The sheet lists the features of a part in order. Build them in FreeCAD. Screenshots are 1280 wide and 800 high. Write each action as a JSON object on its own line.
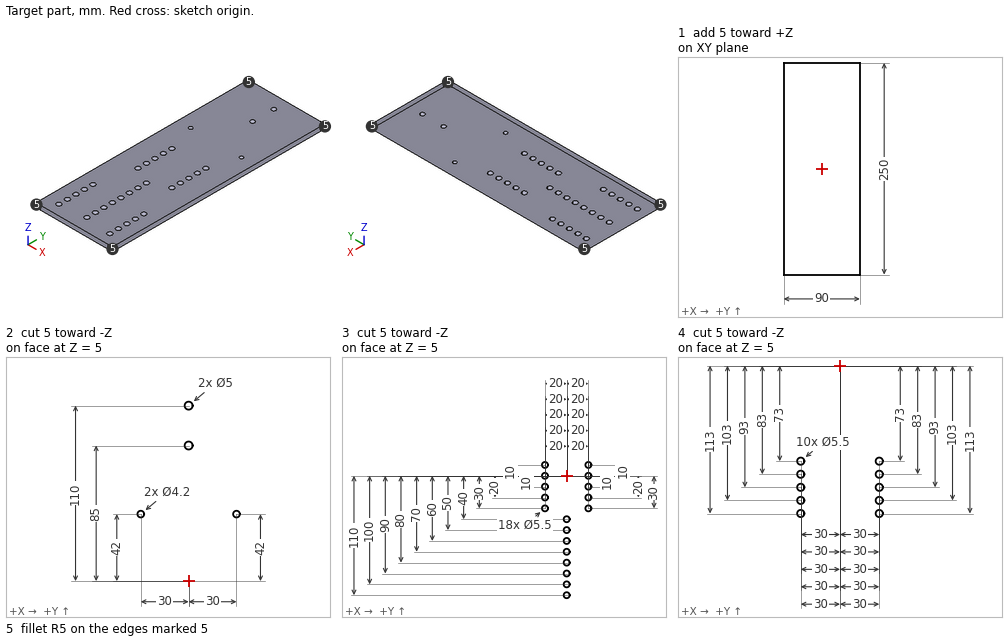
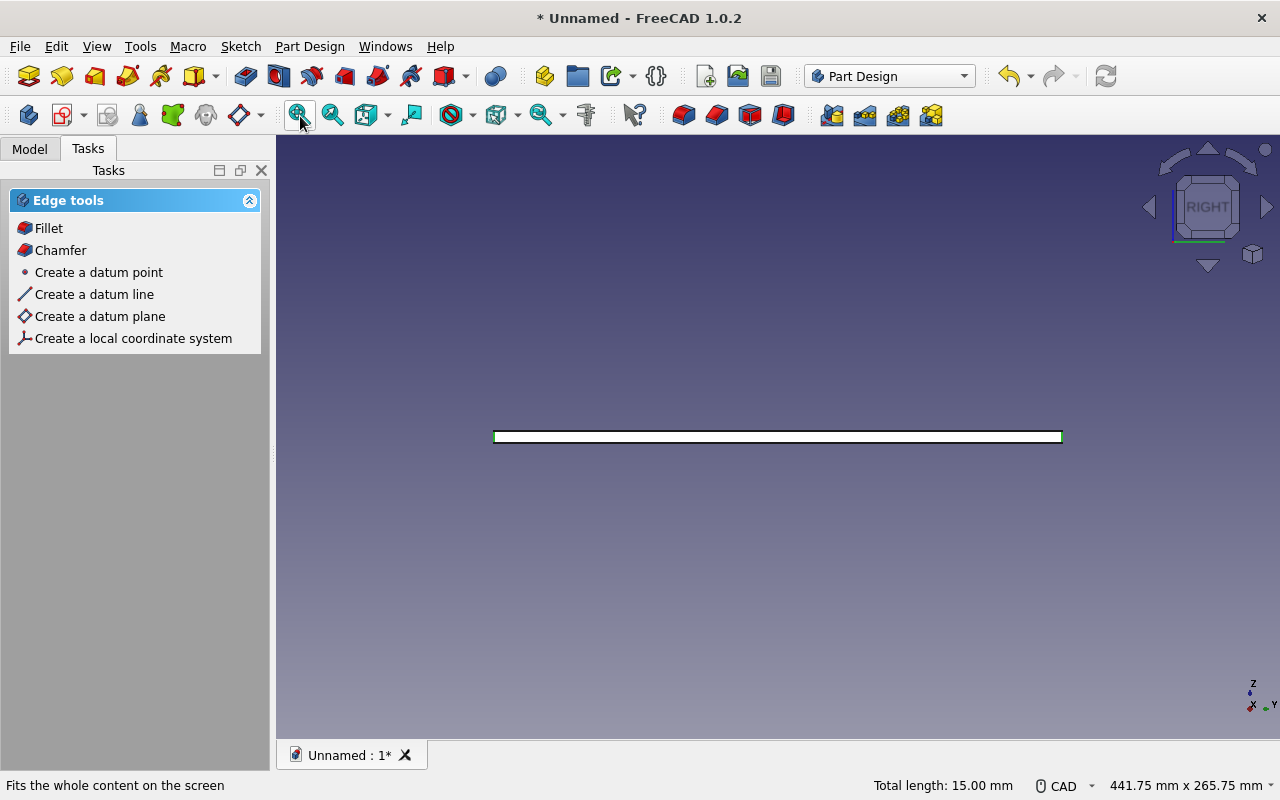
{"action": "key", "text": "5"}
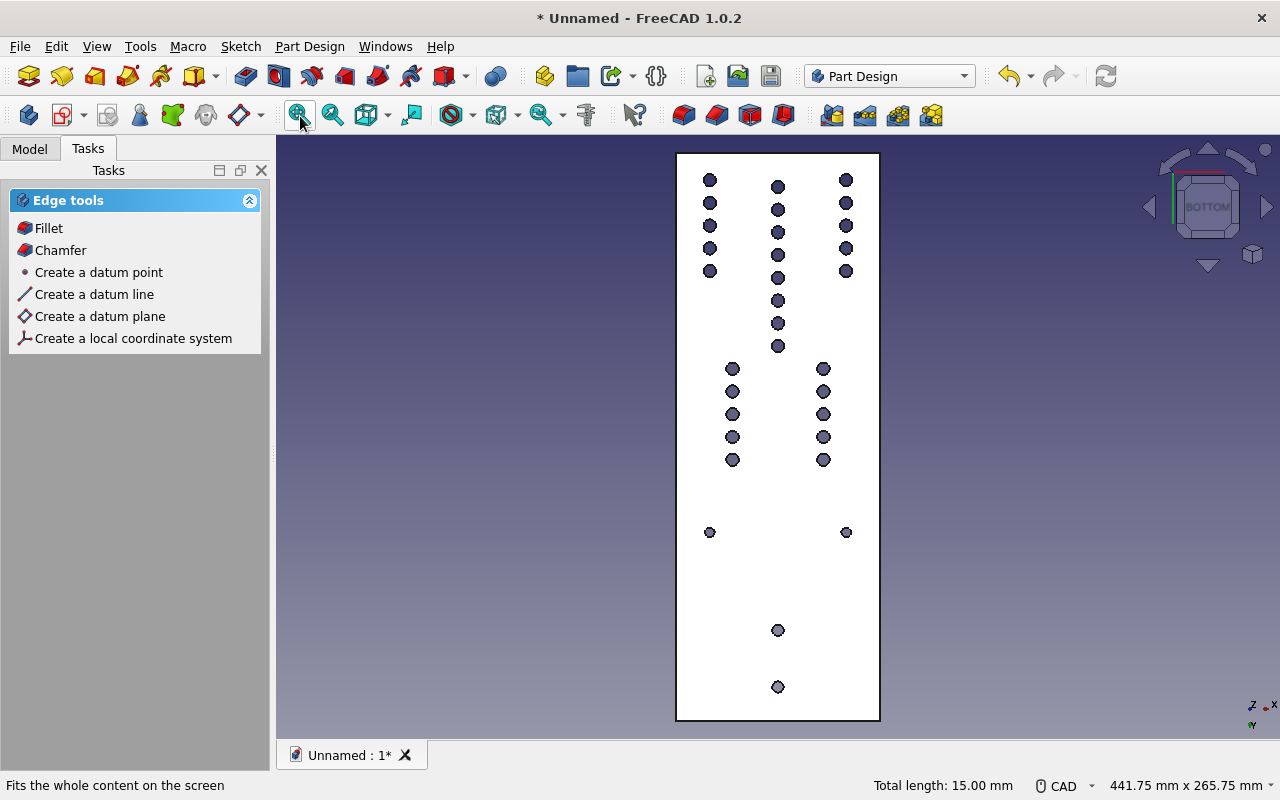
{"action": "key", "text": "4"}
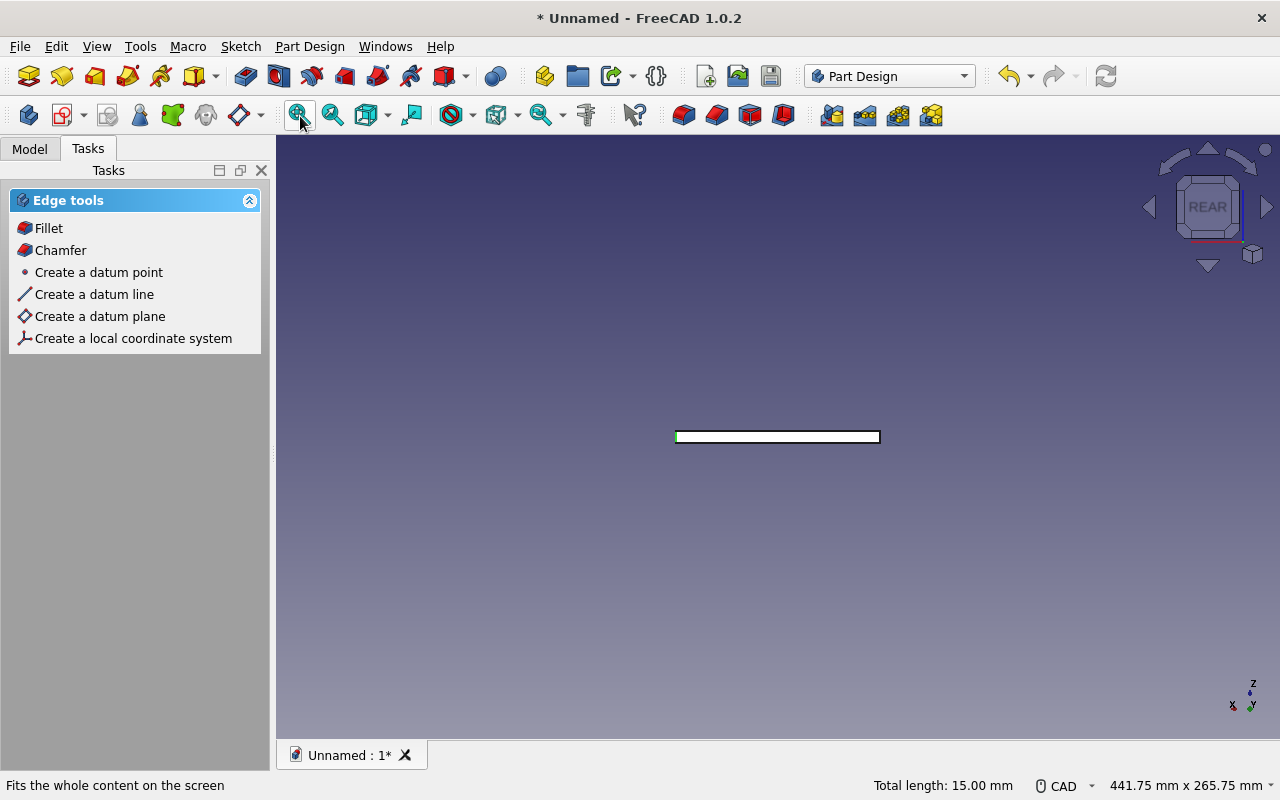
{"action": "key", "text": "v f"}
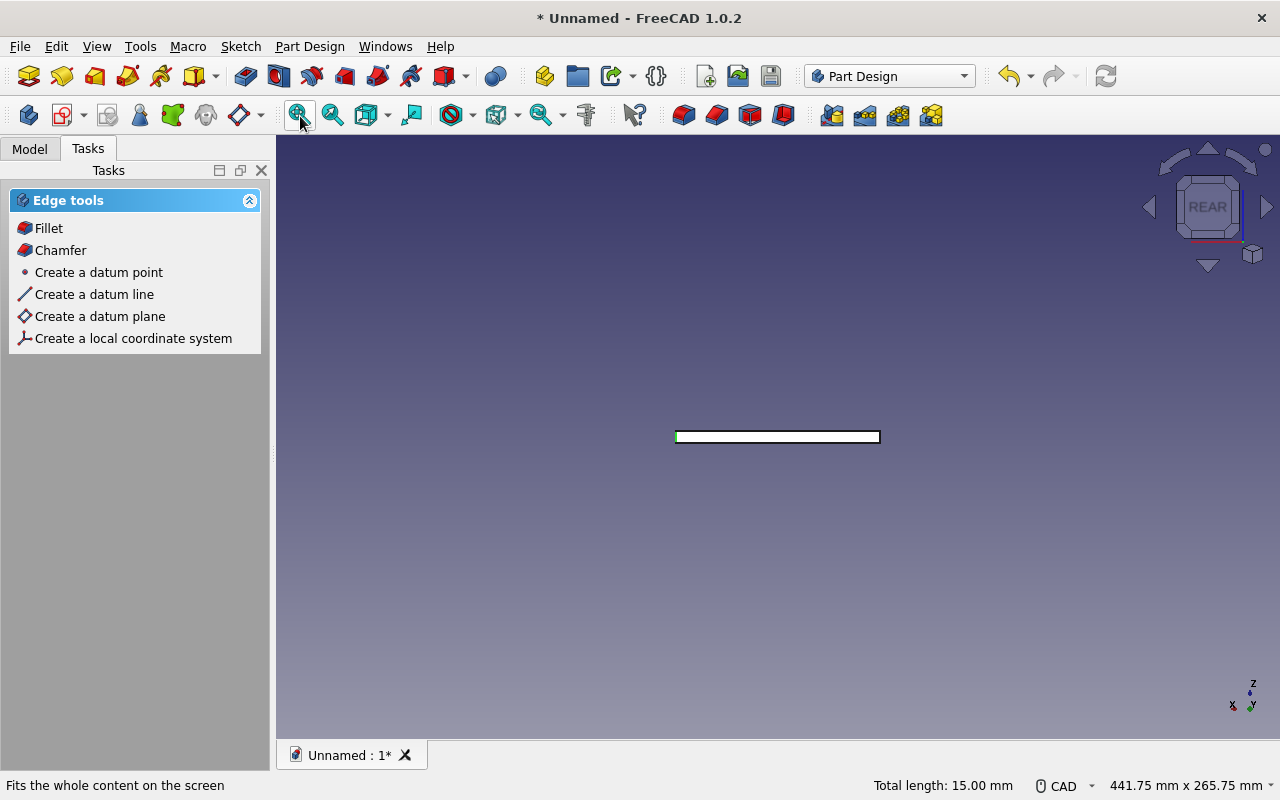
{"action": "scroll", "coordinate": [880, 436], "scroll_direction": "up", "scroll_amount": 7}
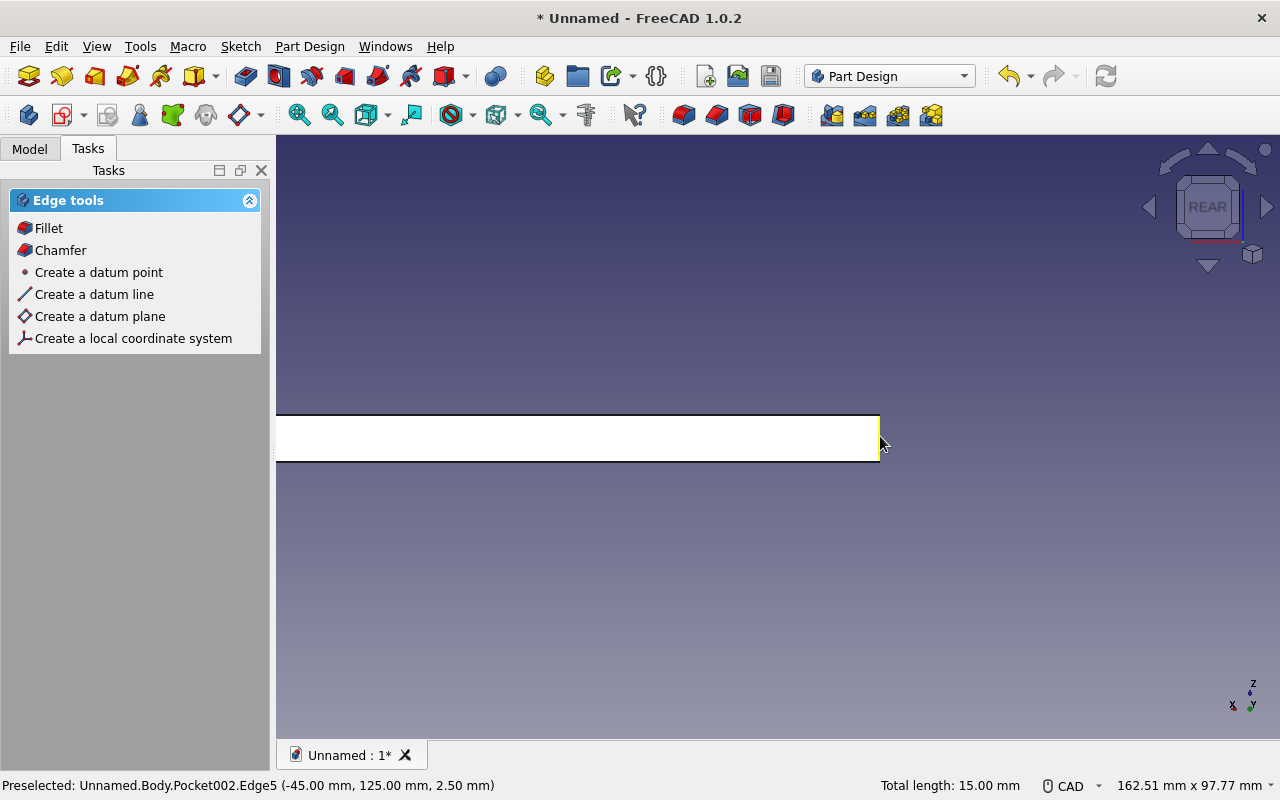
{"action": "left_click", "coordinate": [879, 438], "text": "ctrl"}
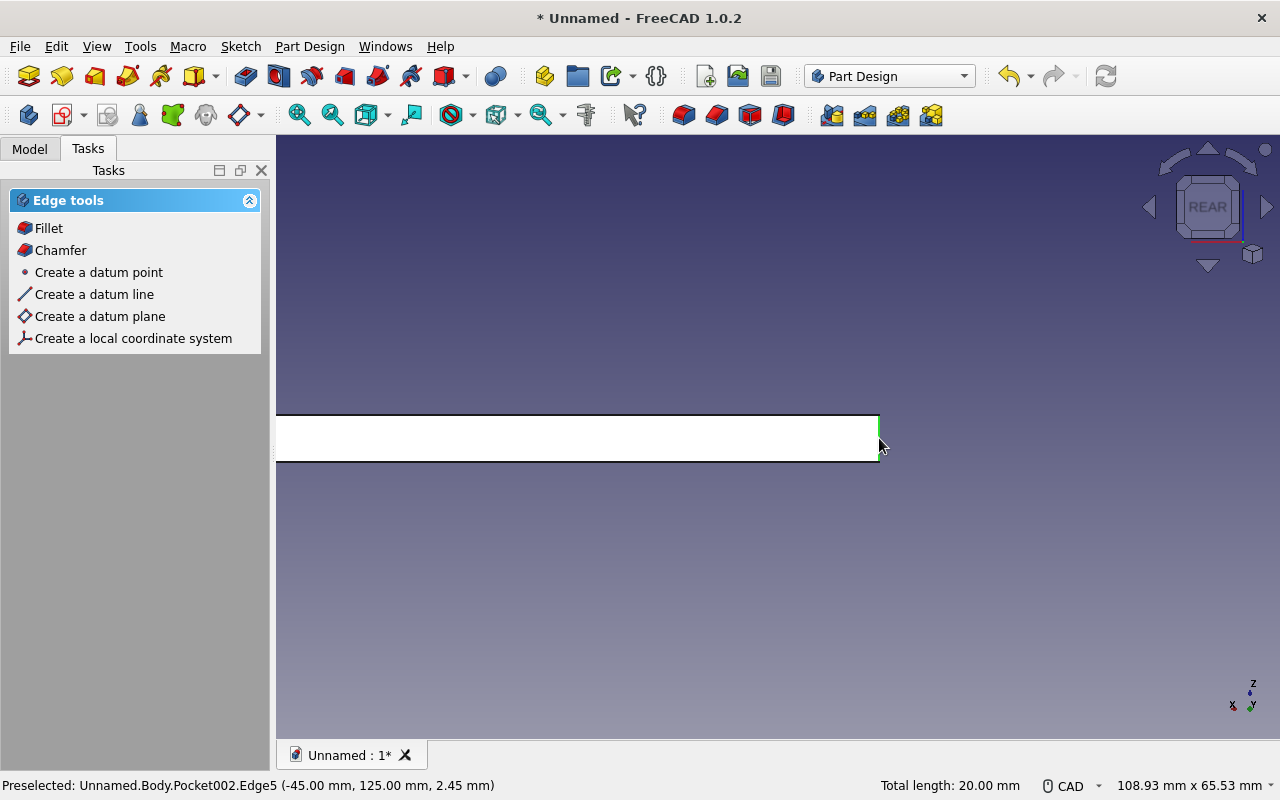
{"action": "left_click", "coordinate": [684, 116]}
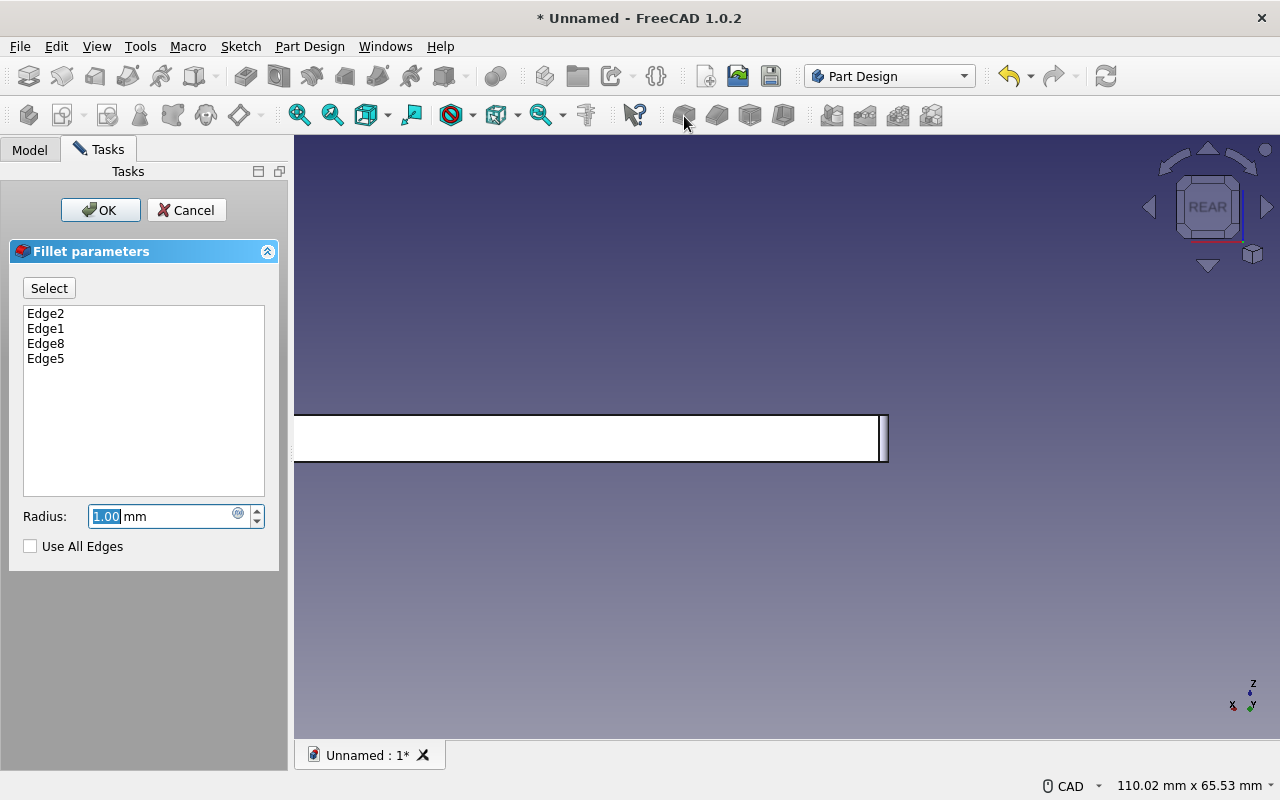
{"action": "type", "text": "5"}
{"action": "key", "text": "Tab"}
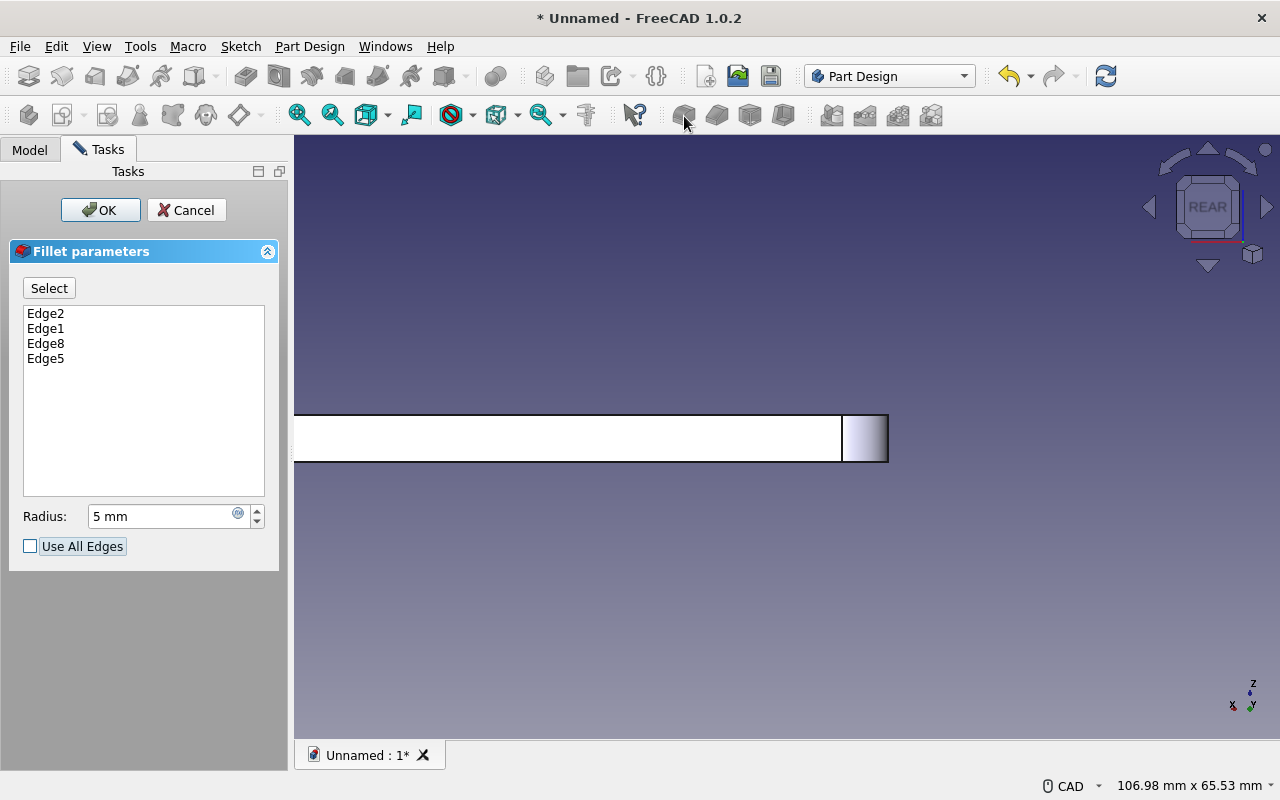
{"action": "left_click", "coordinate": [101, 210]}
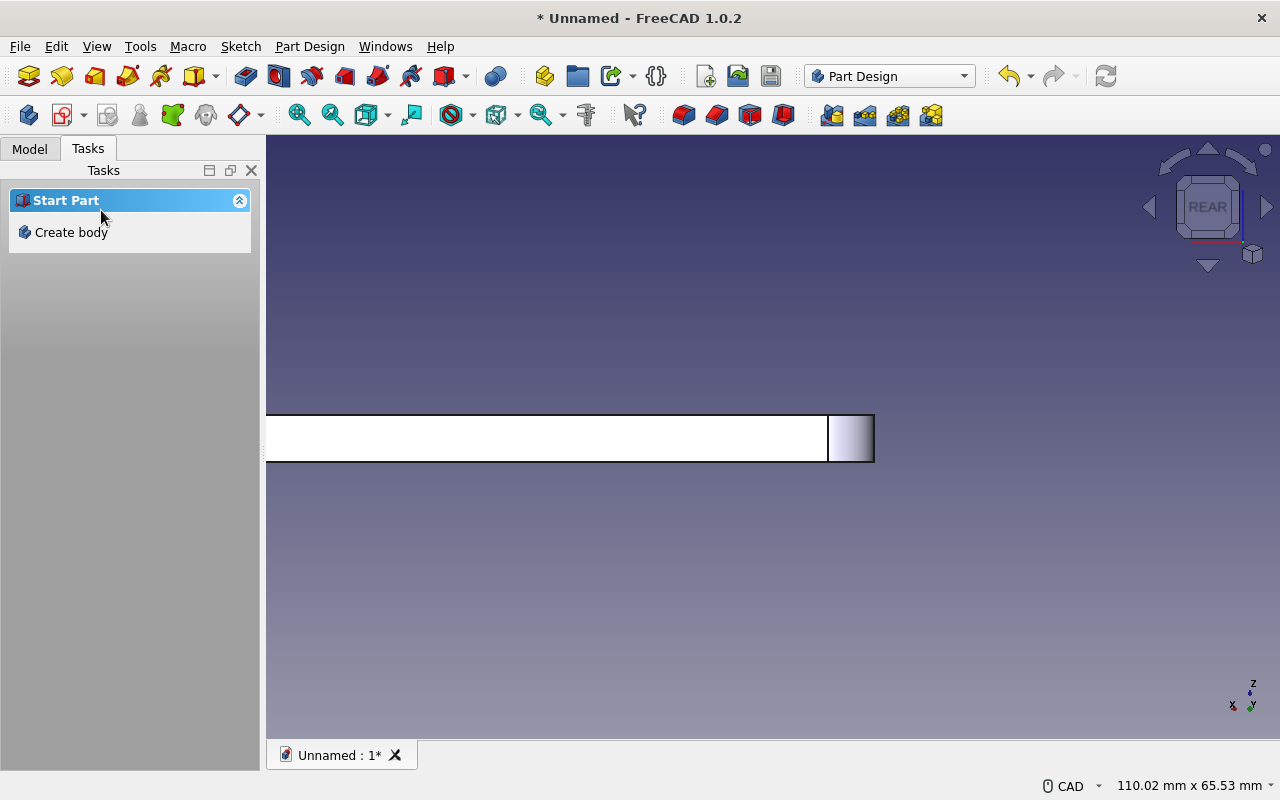
{"action": "key", "text": "0"}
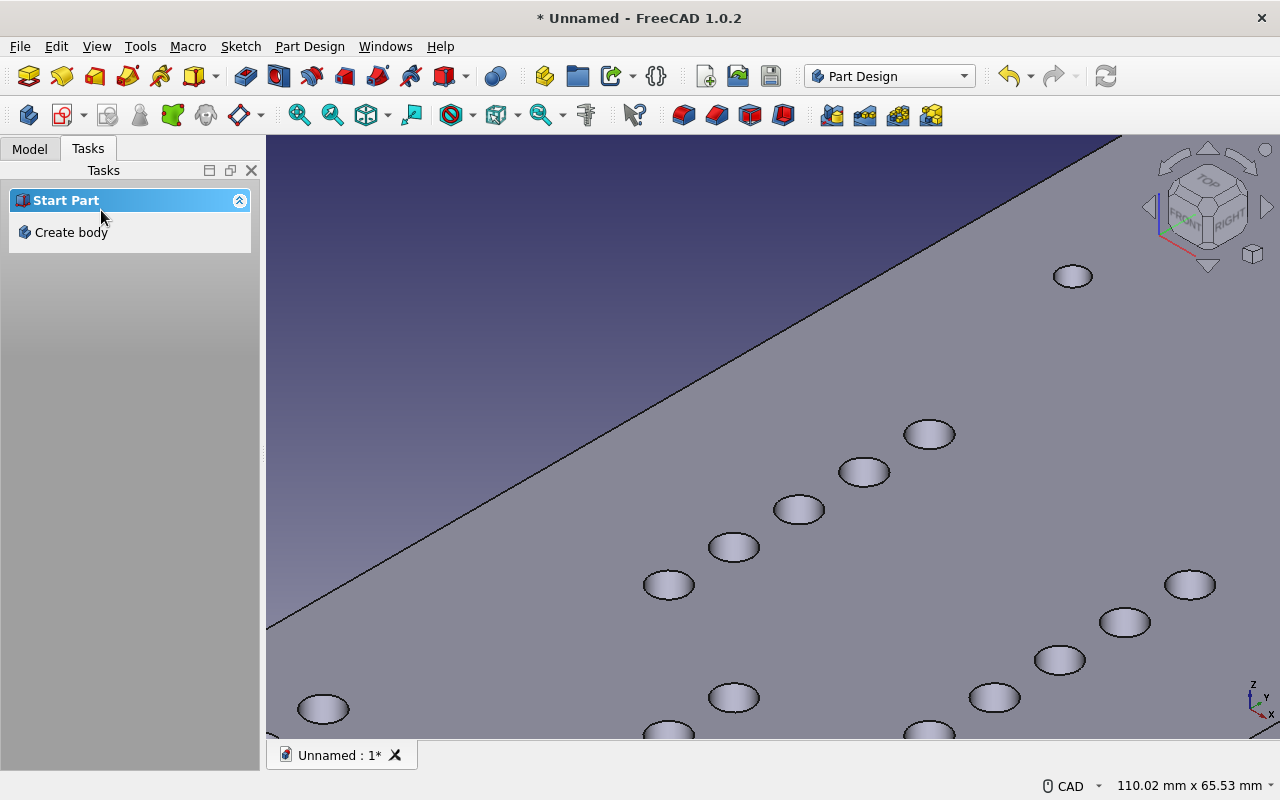
{"action": "key", "text": "v f"}